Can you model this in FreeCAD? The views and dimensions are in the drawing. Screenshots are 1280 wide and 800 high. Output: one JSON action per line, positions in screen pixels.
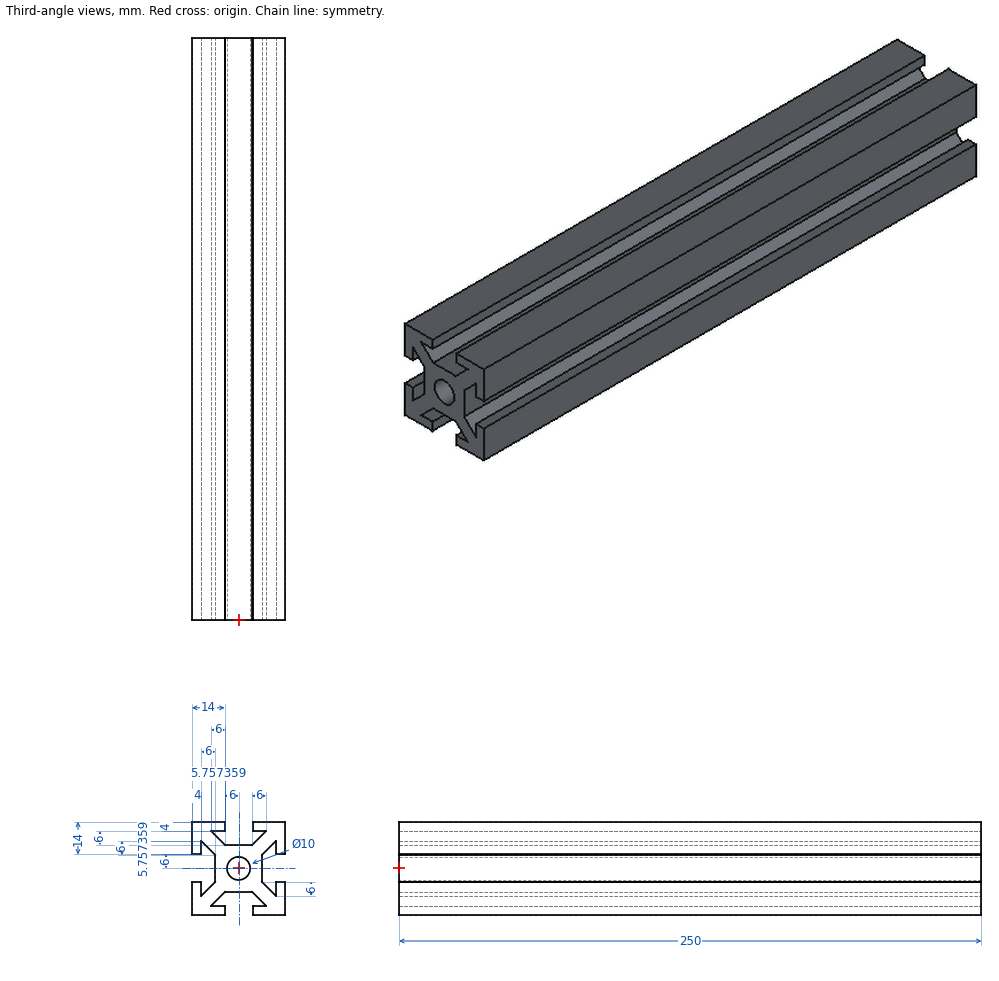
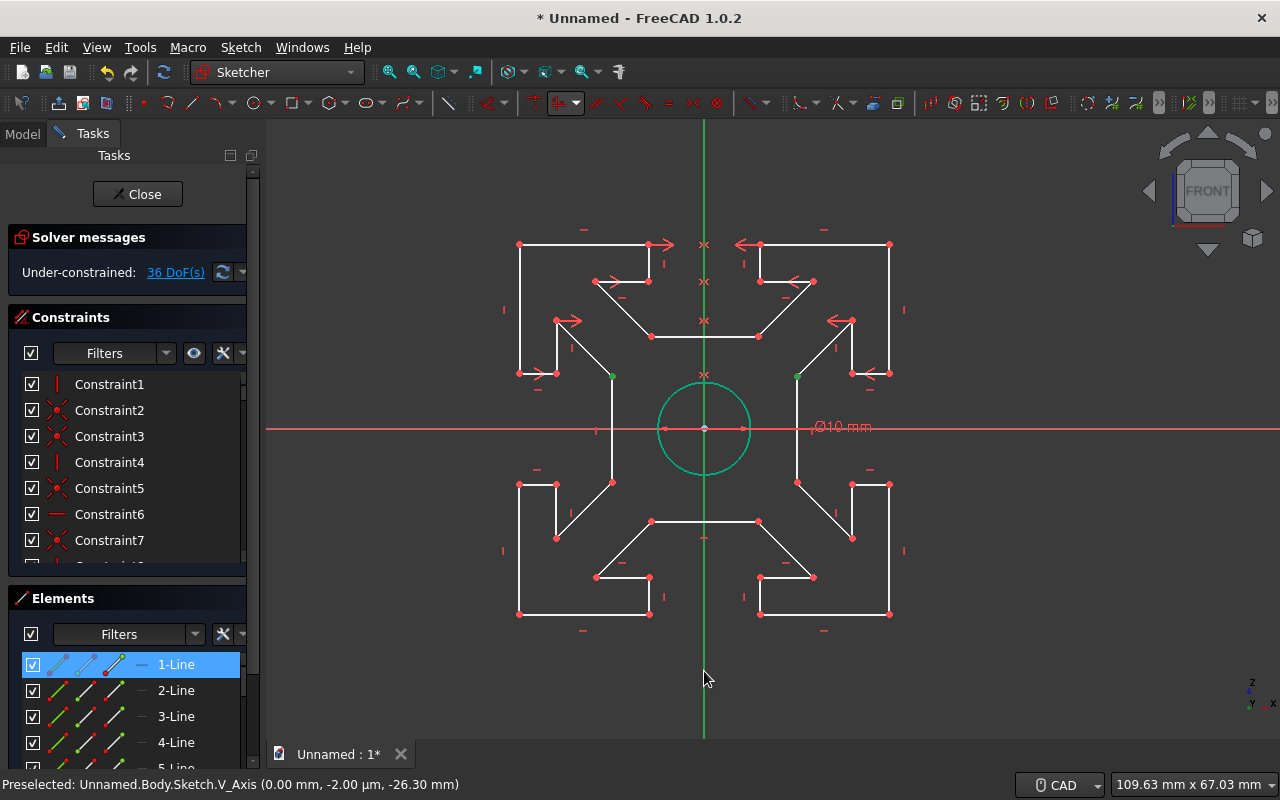
{"action": "left_click", "coordinate": [694, 104]}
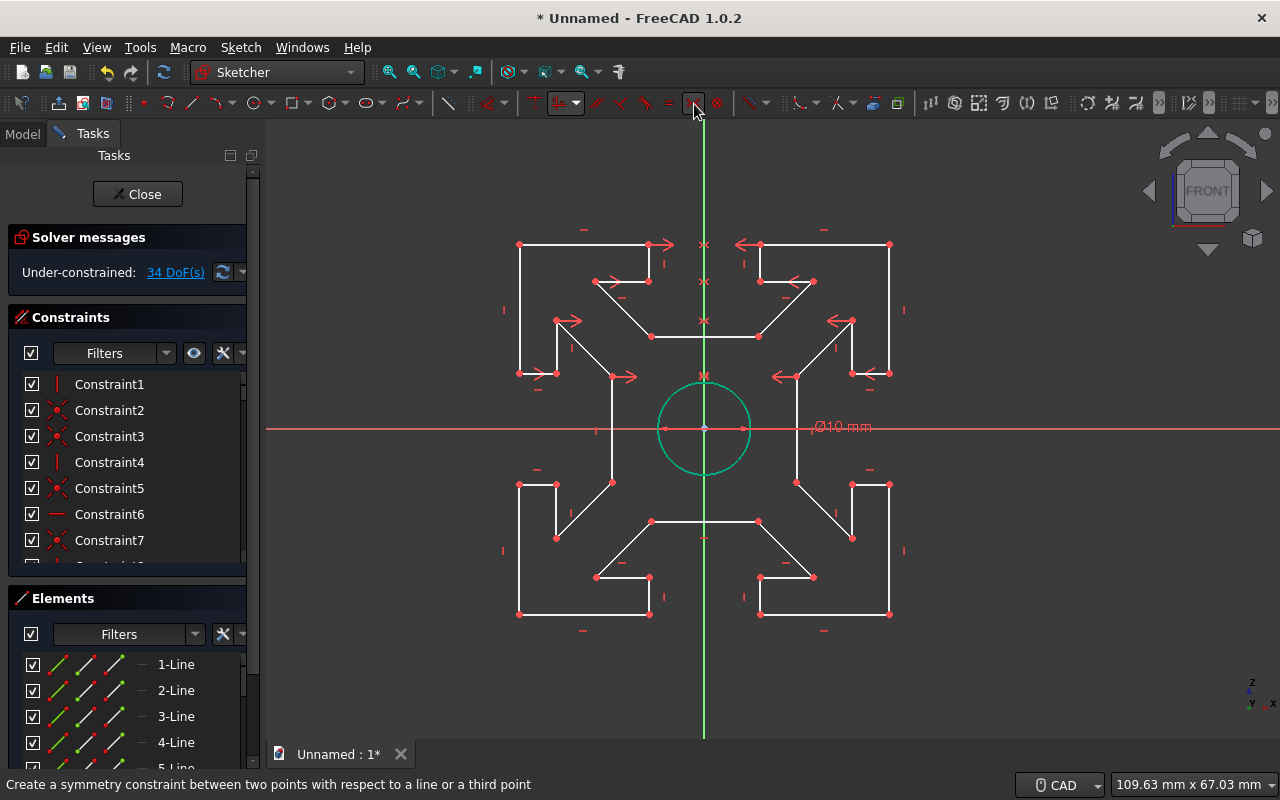
{"action": "left_click", "coordinate": [852, 321]}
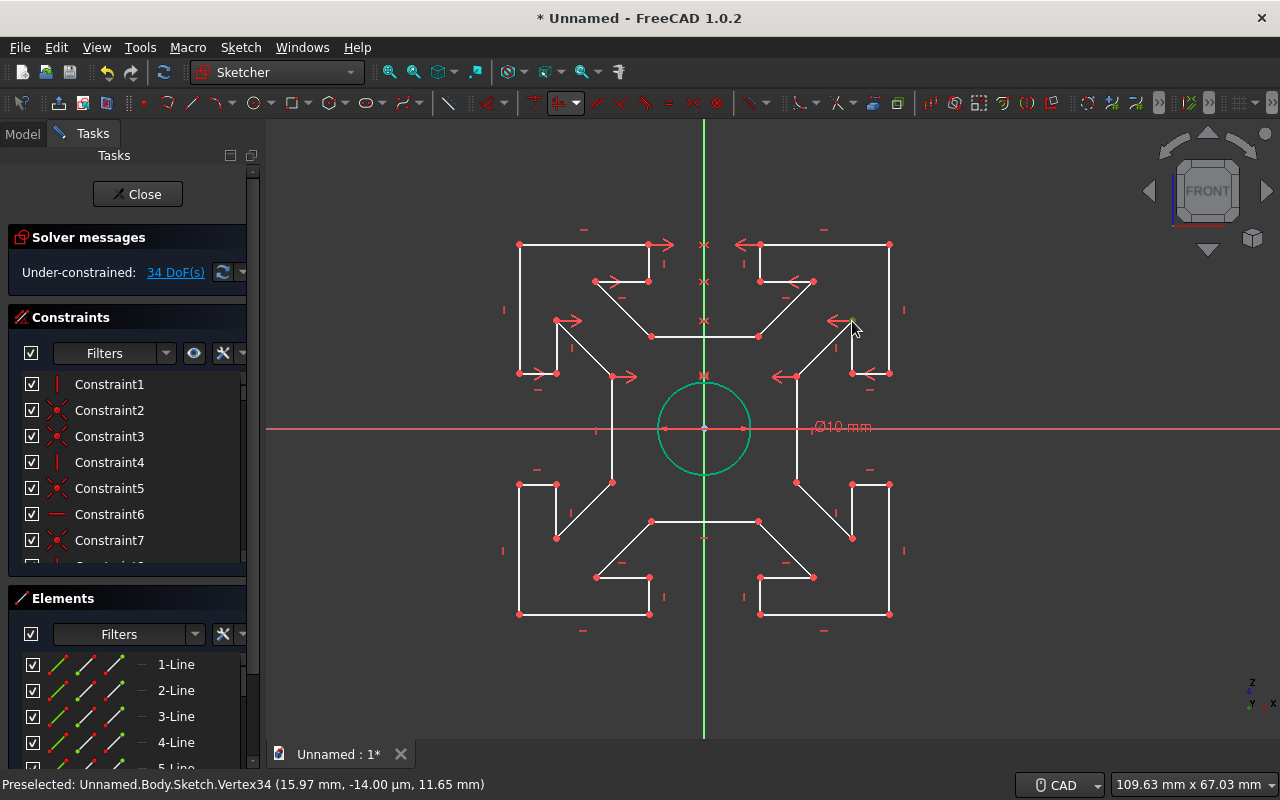
{"action": "left_click", "coordinate": [852, 539]}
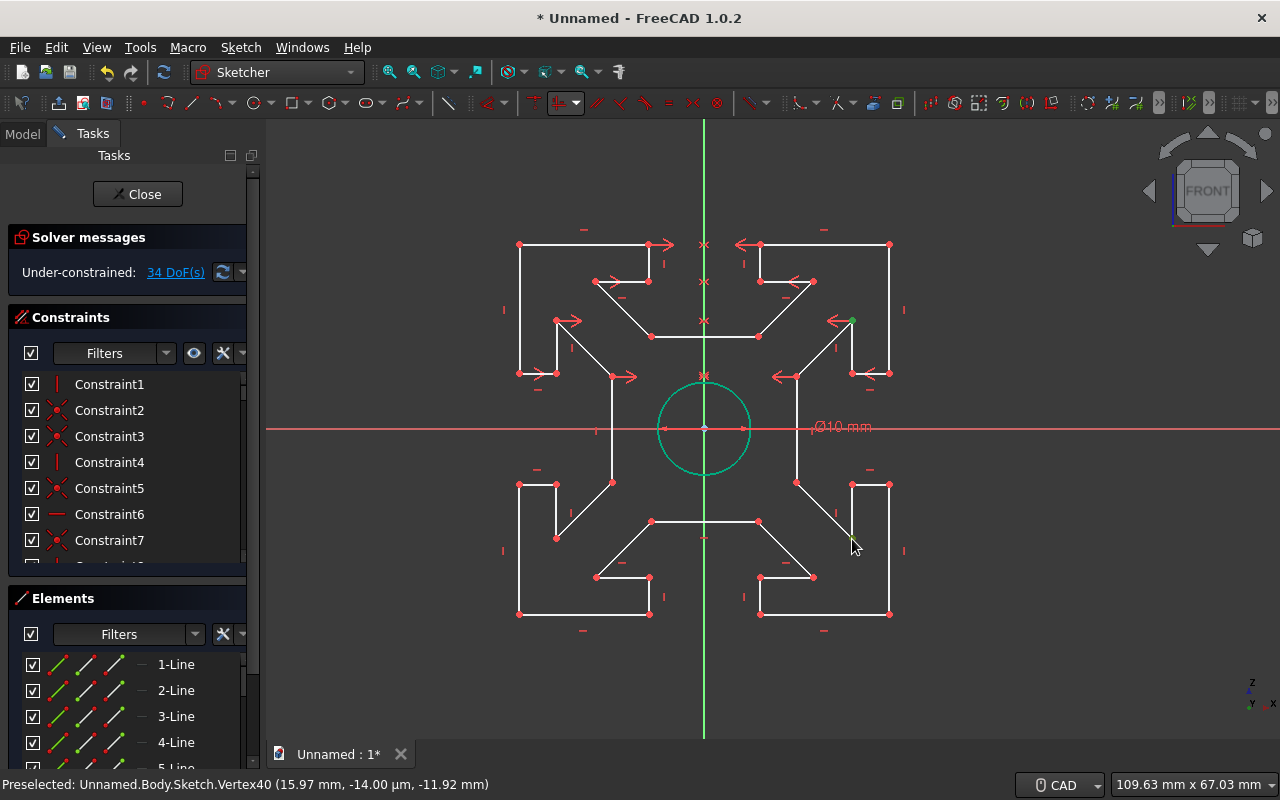
{"action": "left_click", "coordinate": [353, 429]}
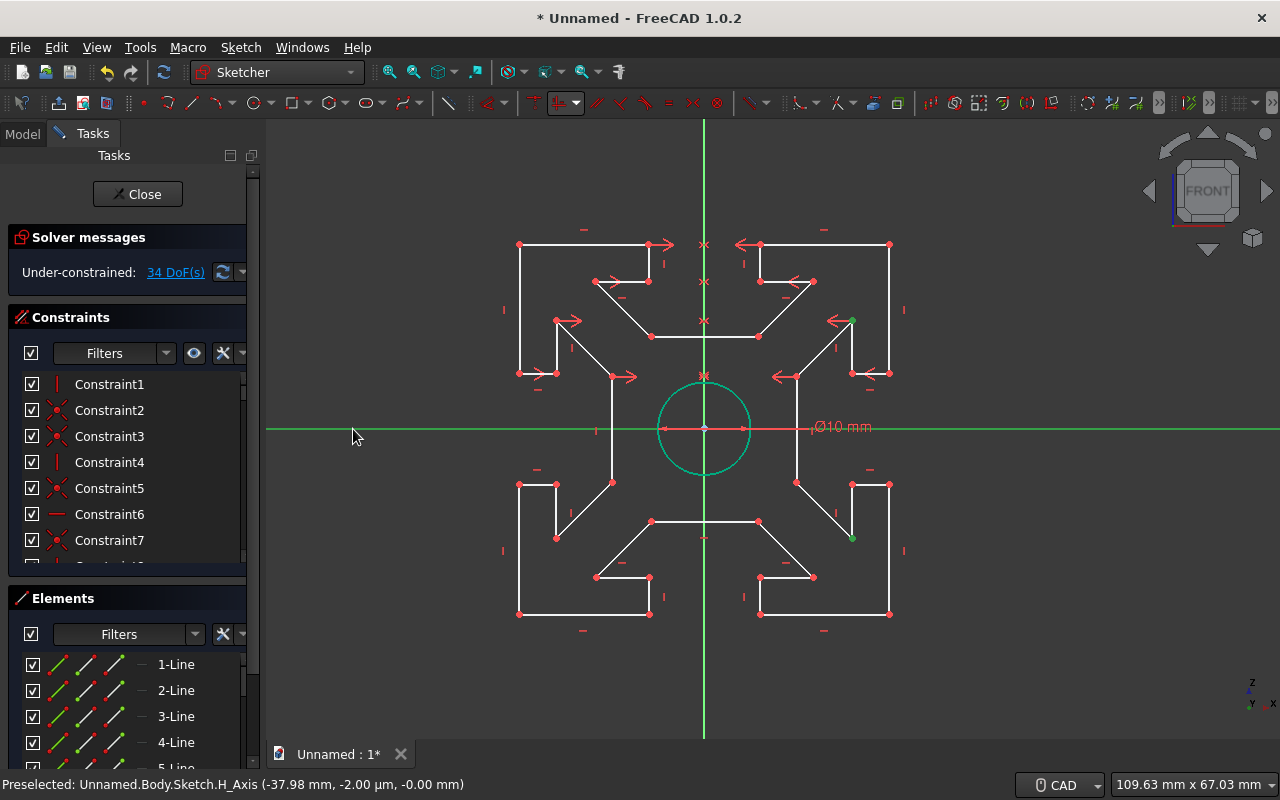
{"action": "left_click", "coordinate": [694, 104]}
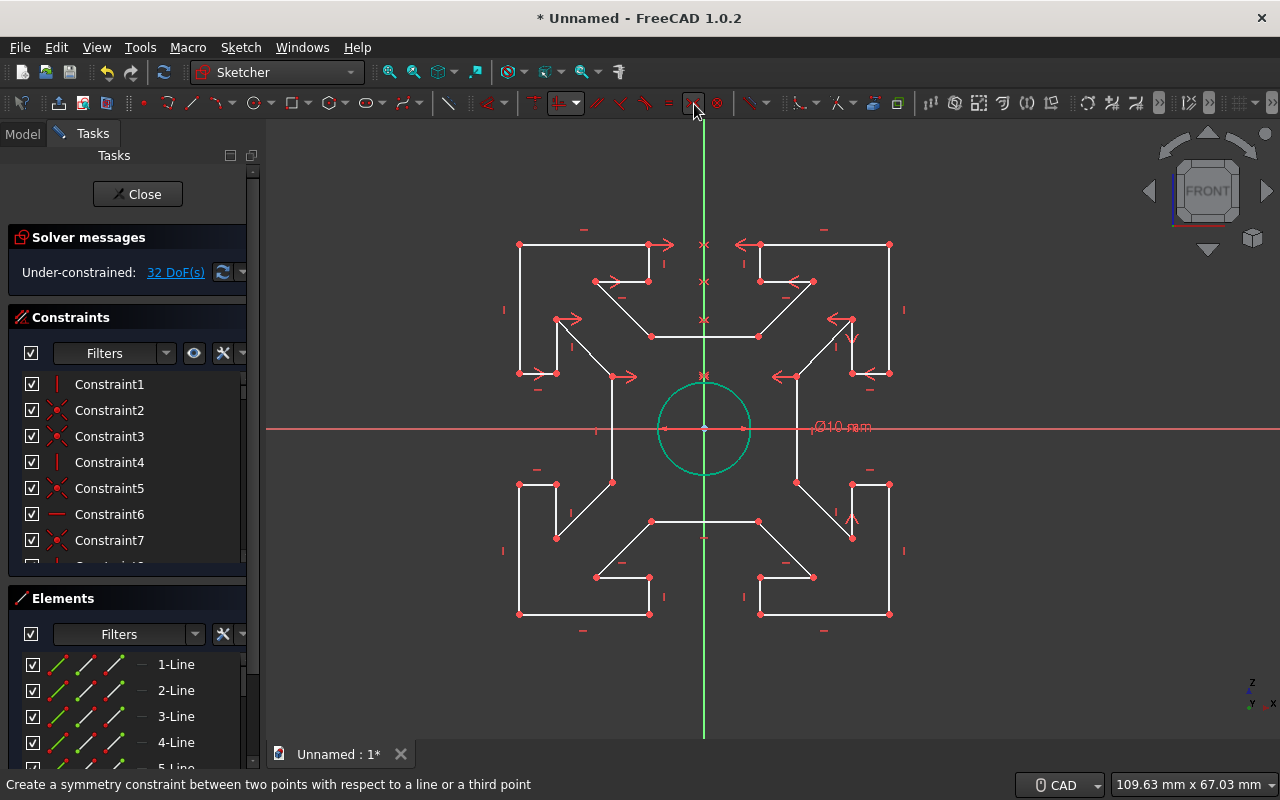
{"action": "left_click", "coordinate": [889, 374]}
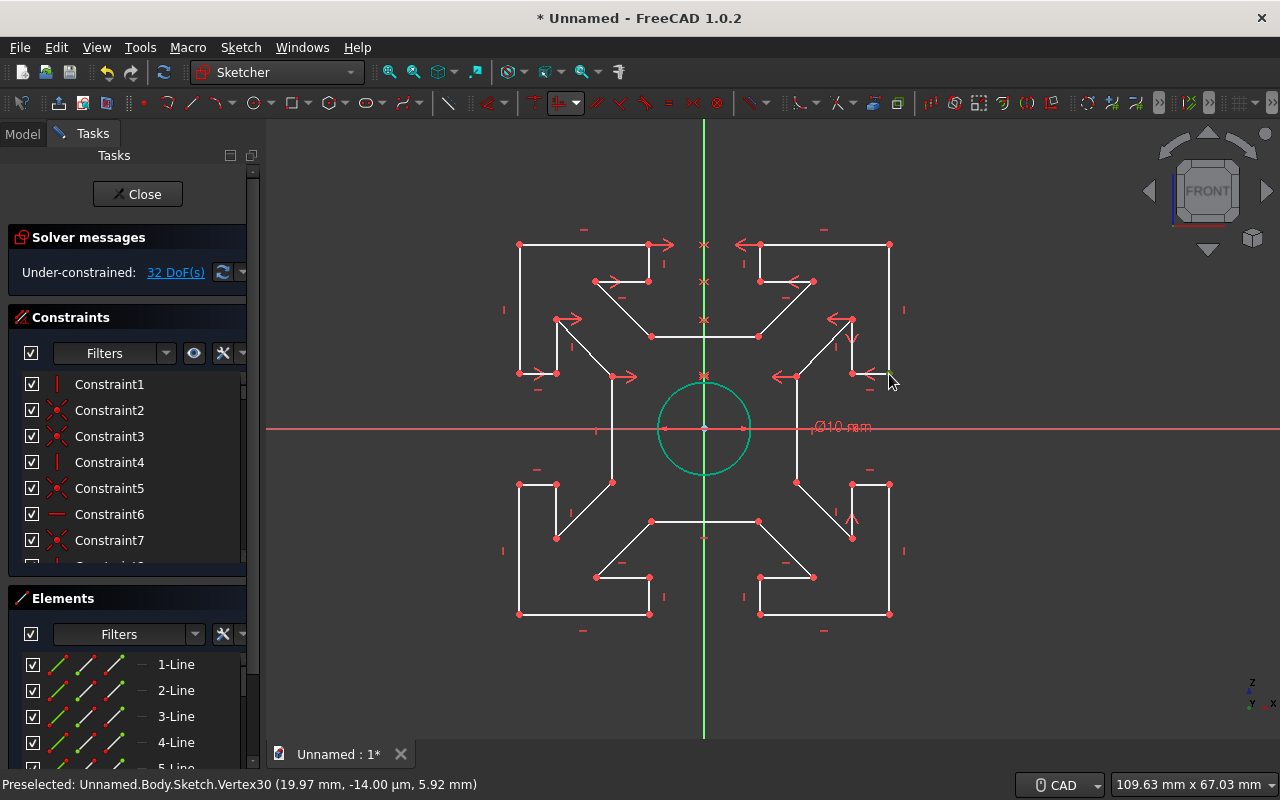
{"action": "left_click", "coordinate": [889, 485]}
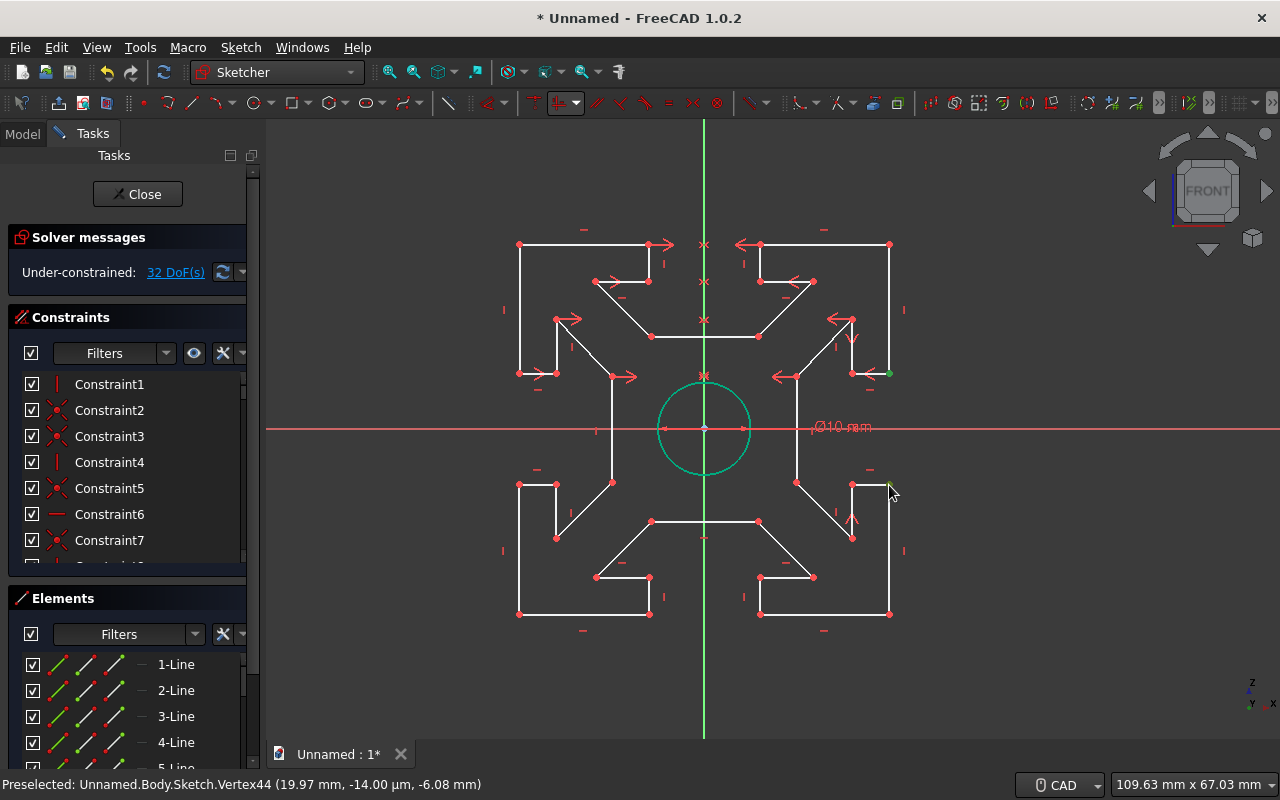
{"action": "left_click", "coordinate": [353, 429]}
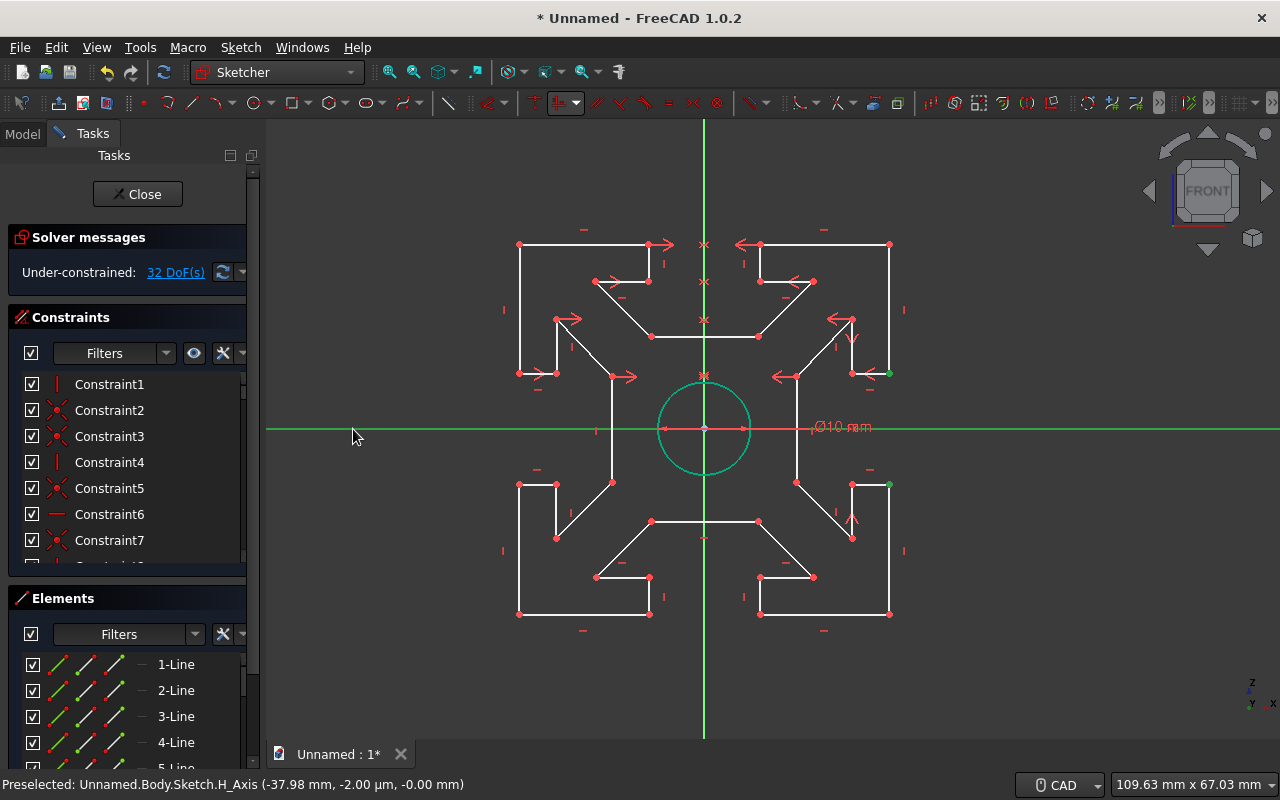
{"action": "left_click", "coordinate": [694, 104]}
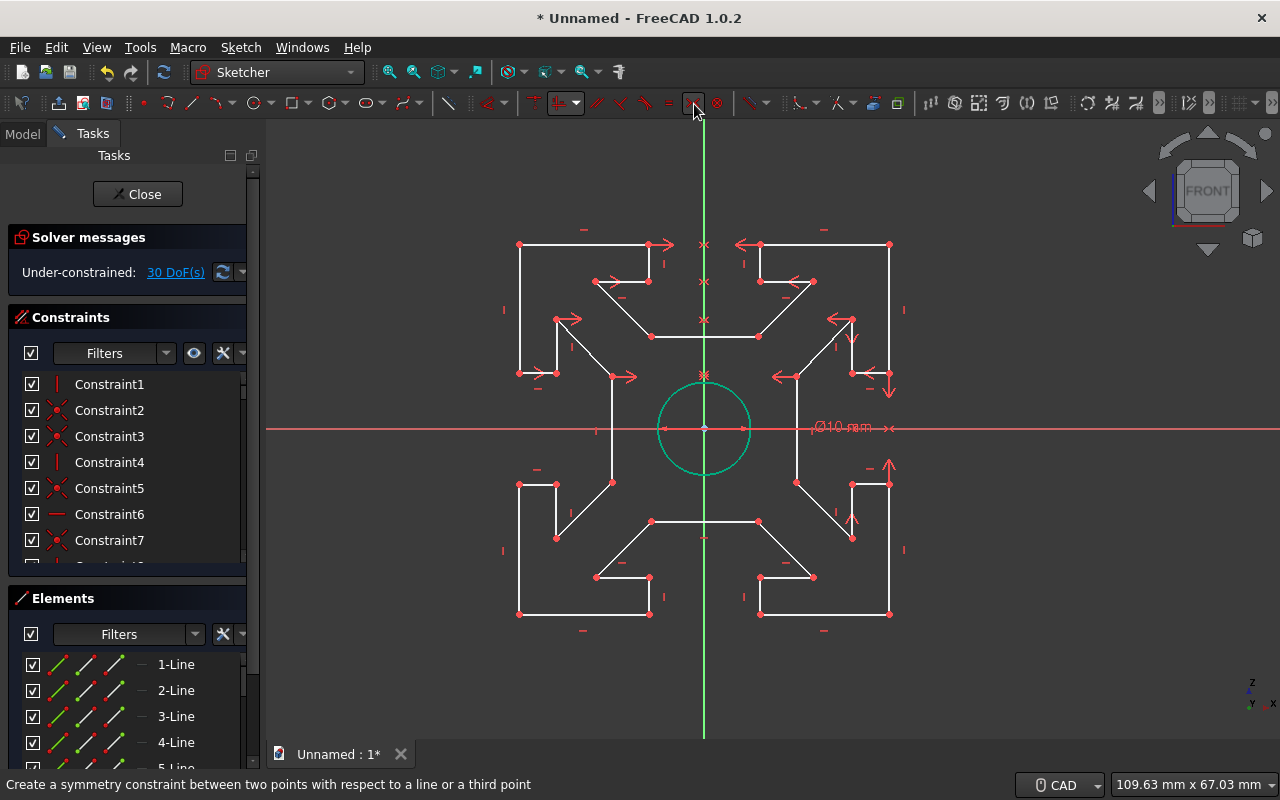
{"action": "left_click", "coordinate": [760, 245]}